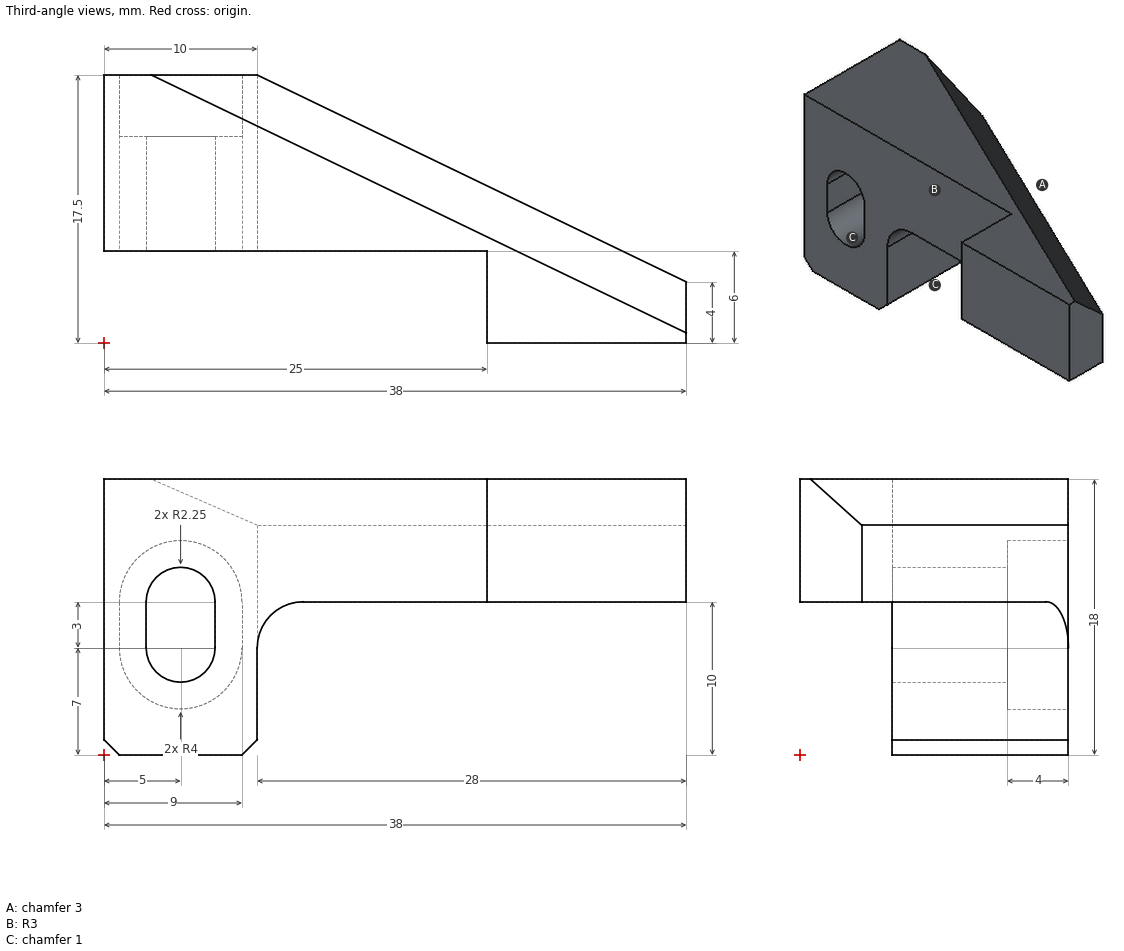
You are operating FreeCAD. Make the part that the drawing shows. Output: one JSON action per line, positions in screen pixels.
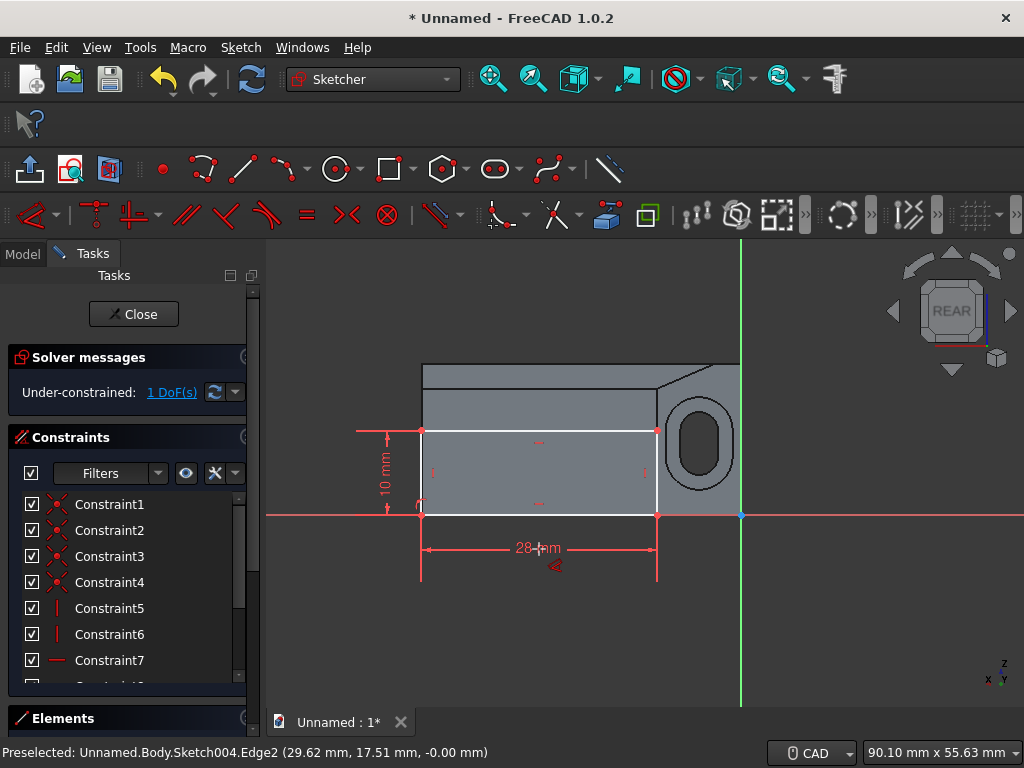
{"action": "left_click", "coordinate": [421, 431]}
{"action": "left_click", "coordinate": [655, 549]}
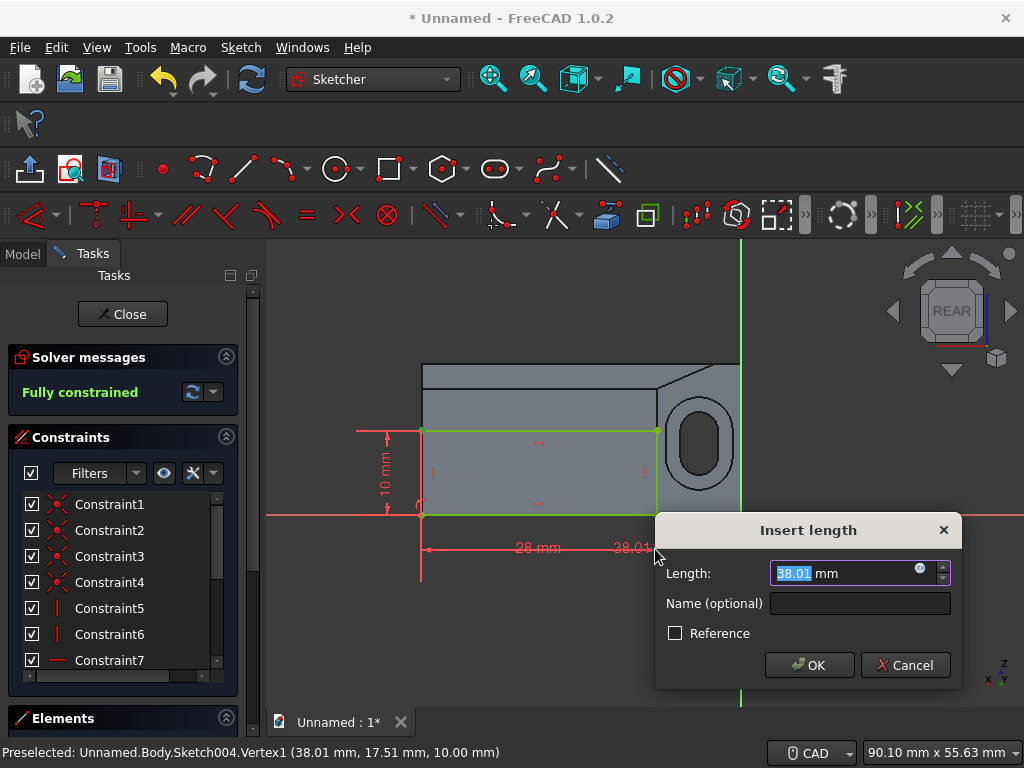
{"action": "type", "text": "38"}
{"action": "key", "text": "Return"}
{"action": "key", "text": "Escape"}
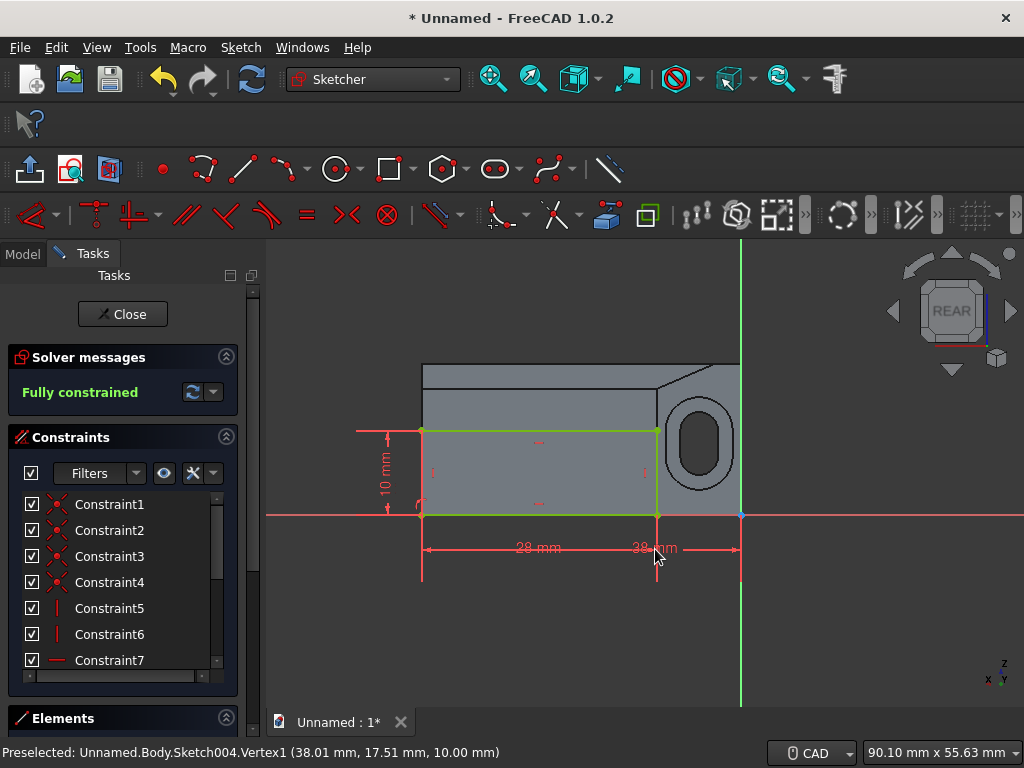
{"action": "left_click", "coordinate": [123, 314]}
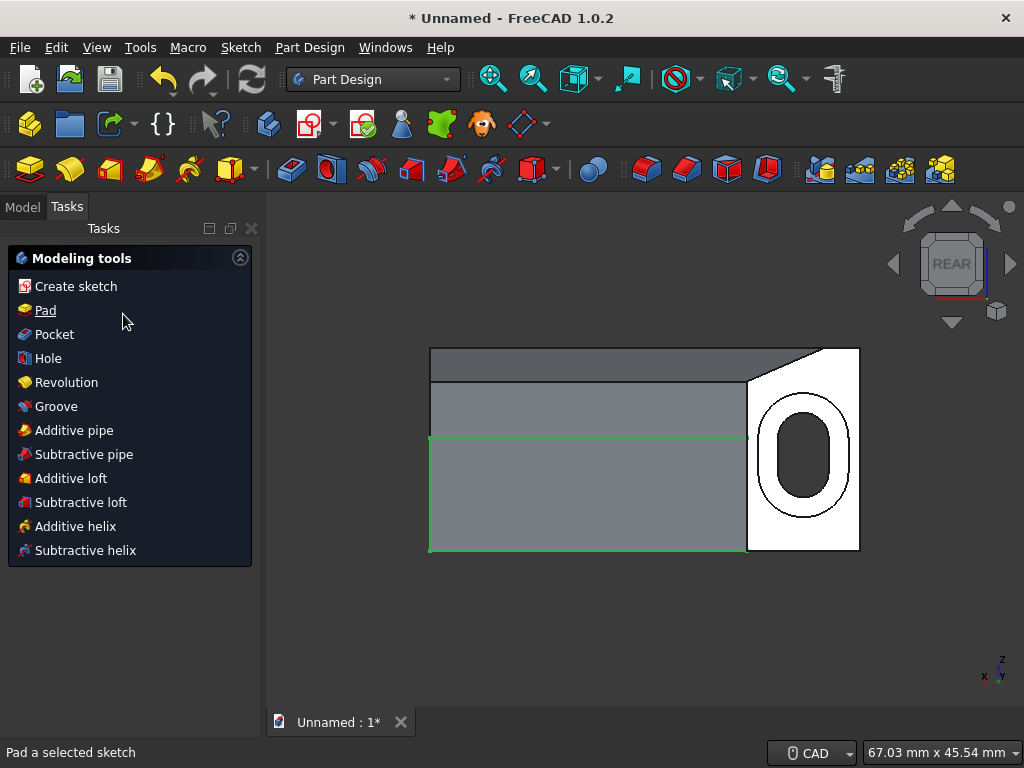
{"action": "left_click", "coordinate": [292, 170]}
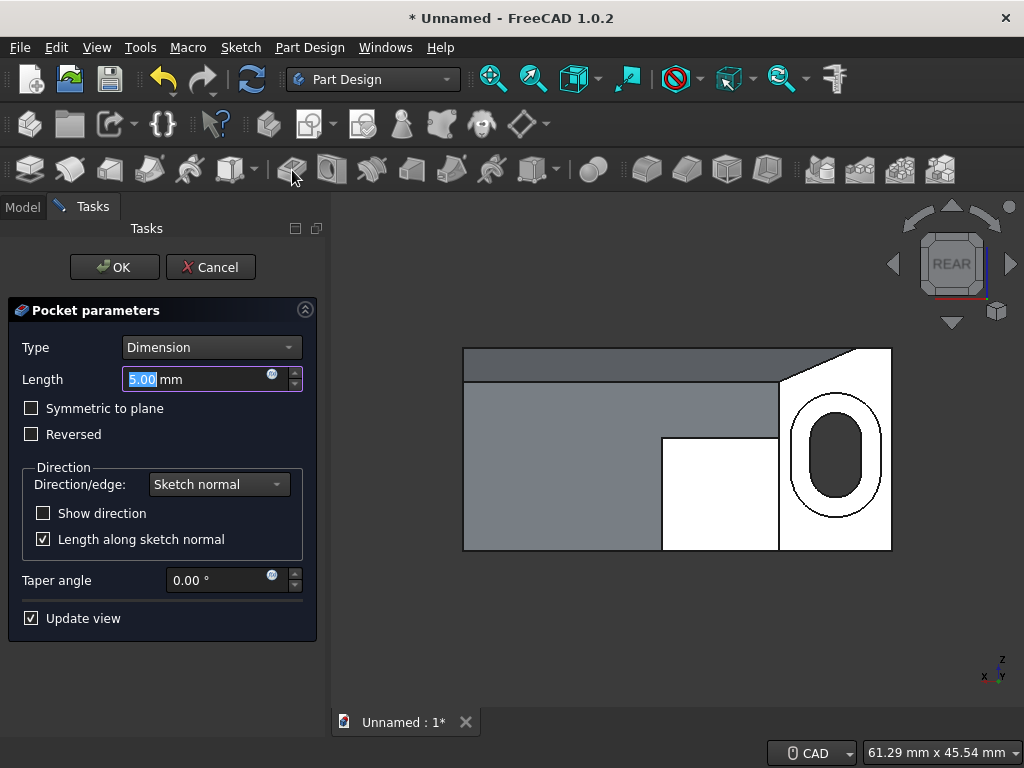
{"action": "left_click", "coordinate": [212, 348]}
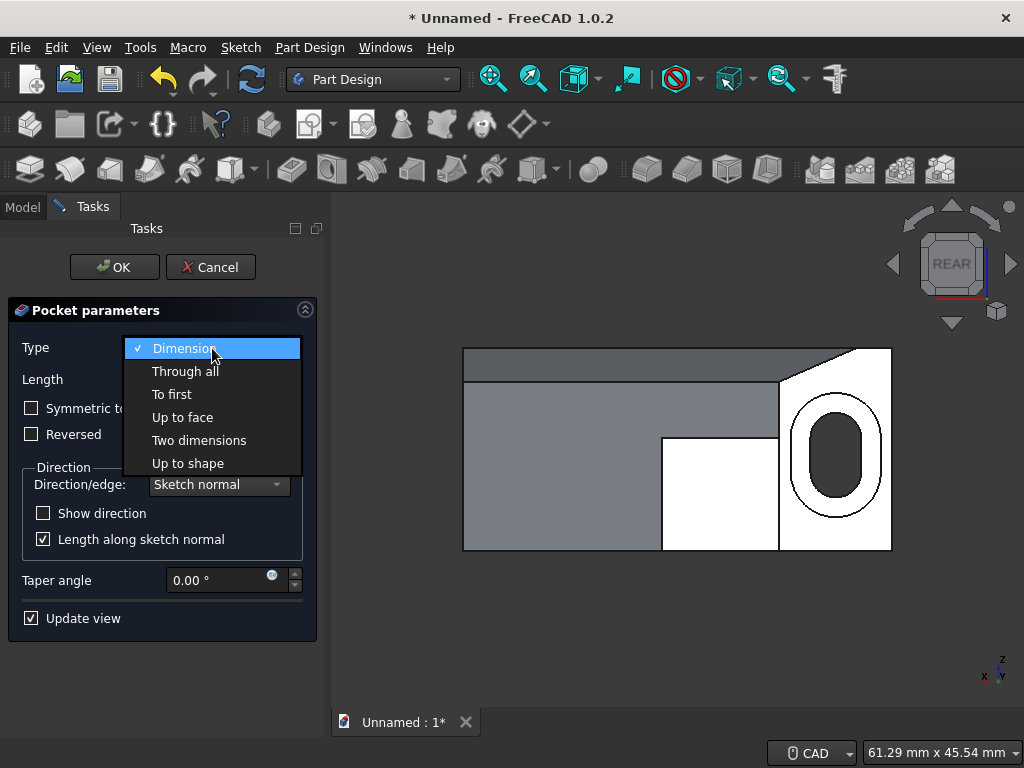
{"action": "left_click", "coordinate": [212, 372]}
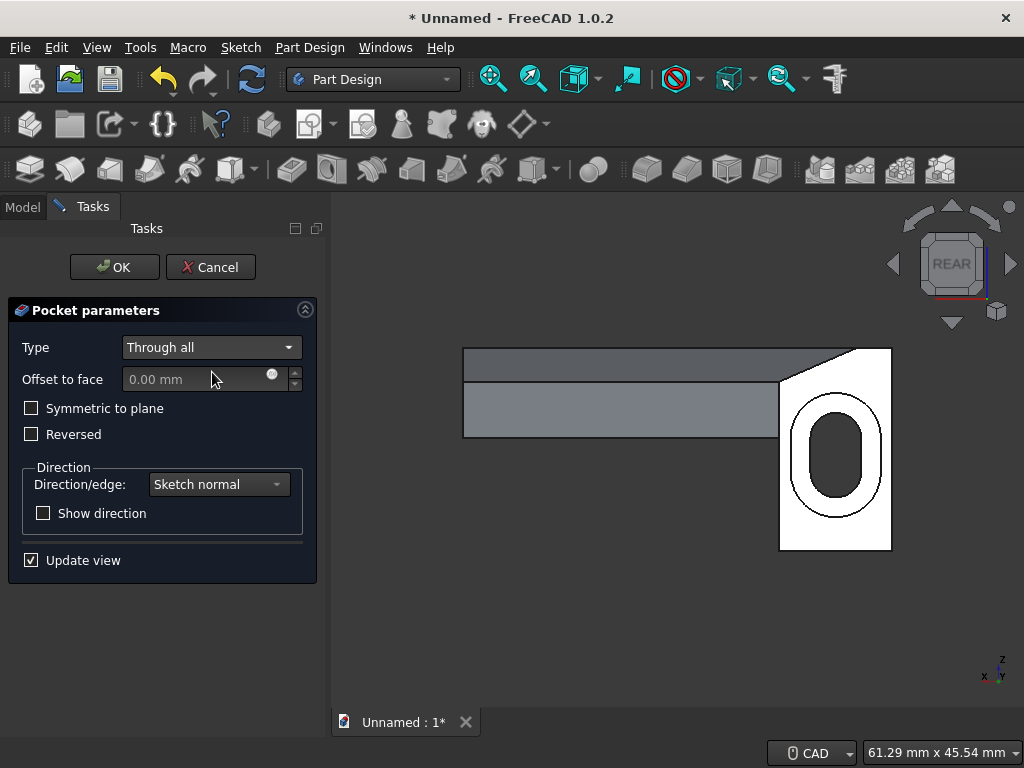
{"action": "left_click", "coordinate": [115, 267]}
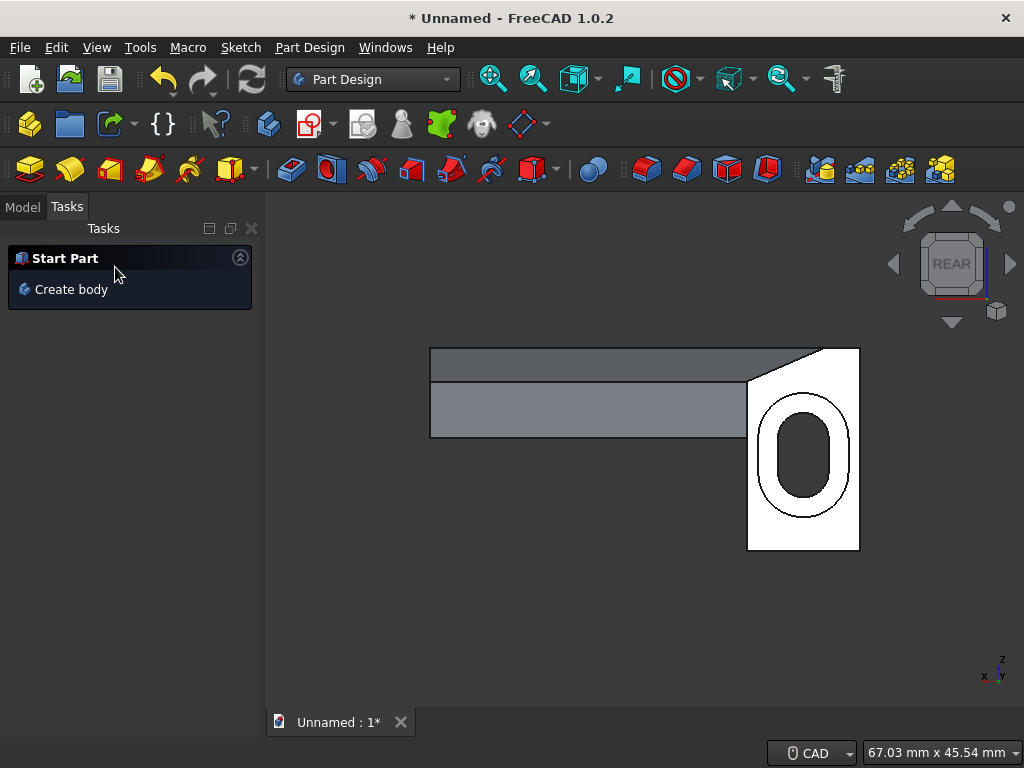
{"action": "key", "text": "0"}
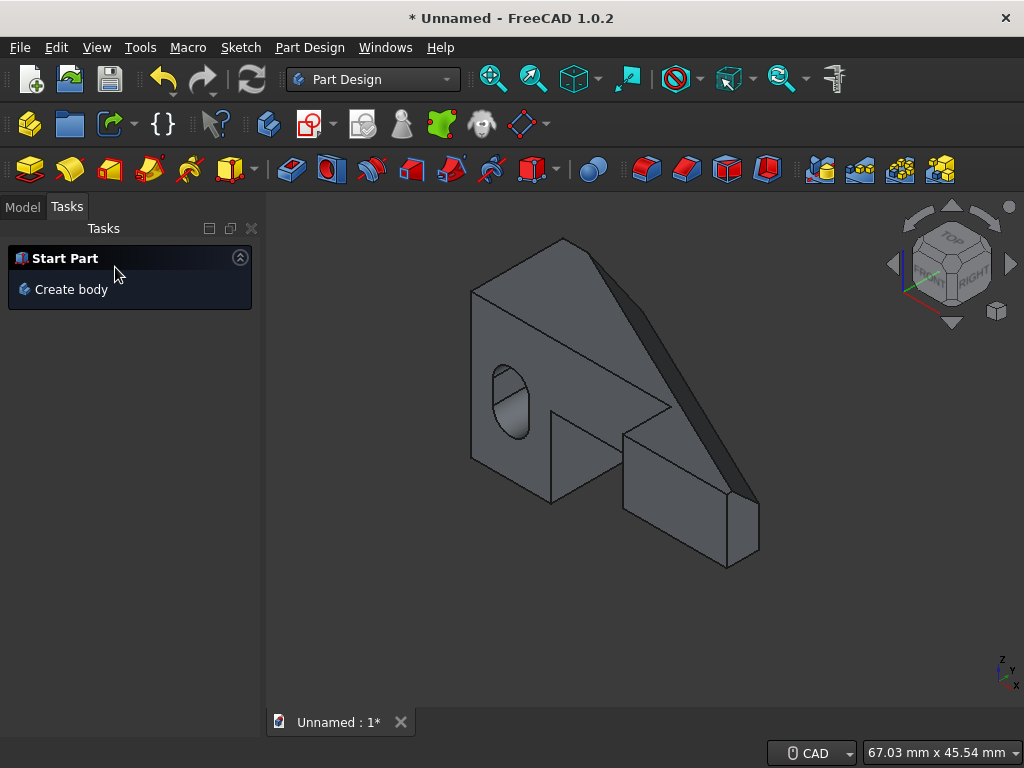
{"action": "key", "text": "2"}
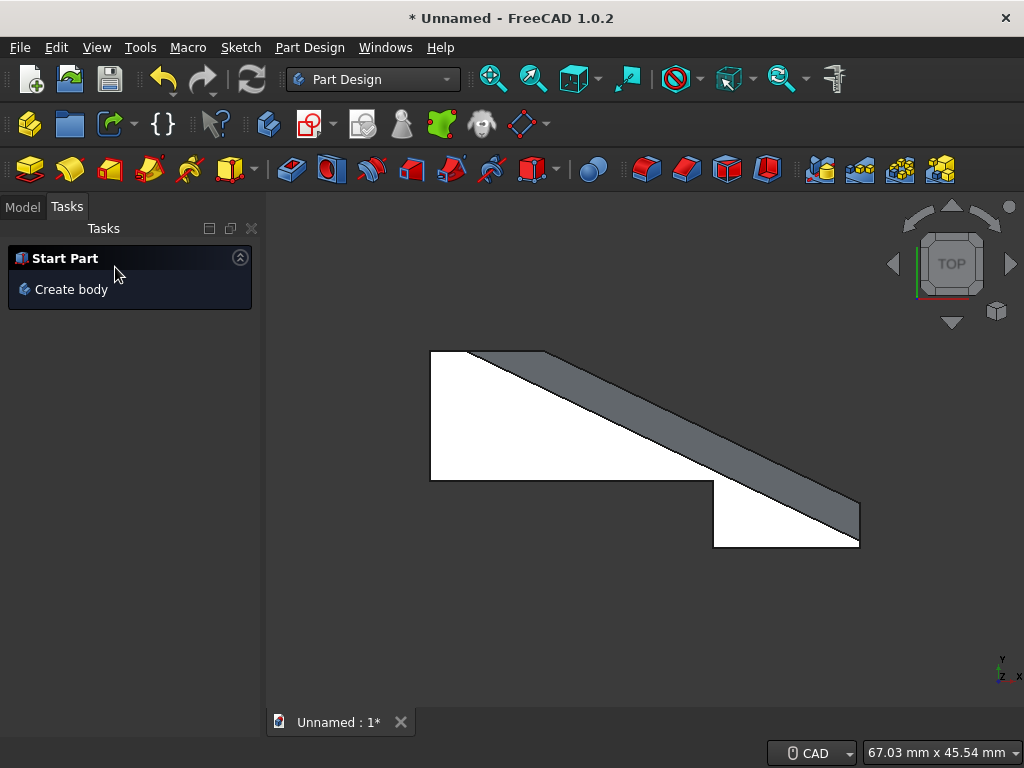
{"action": "key", "text": "1"}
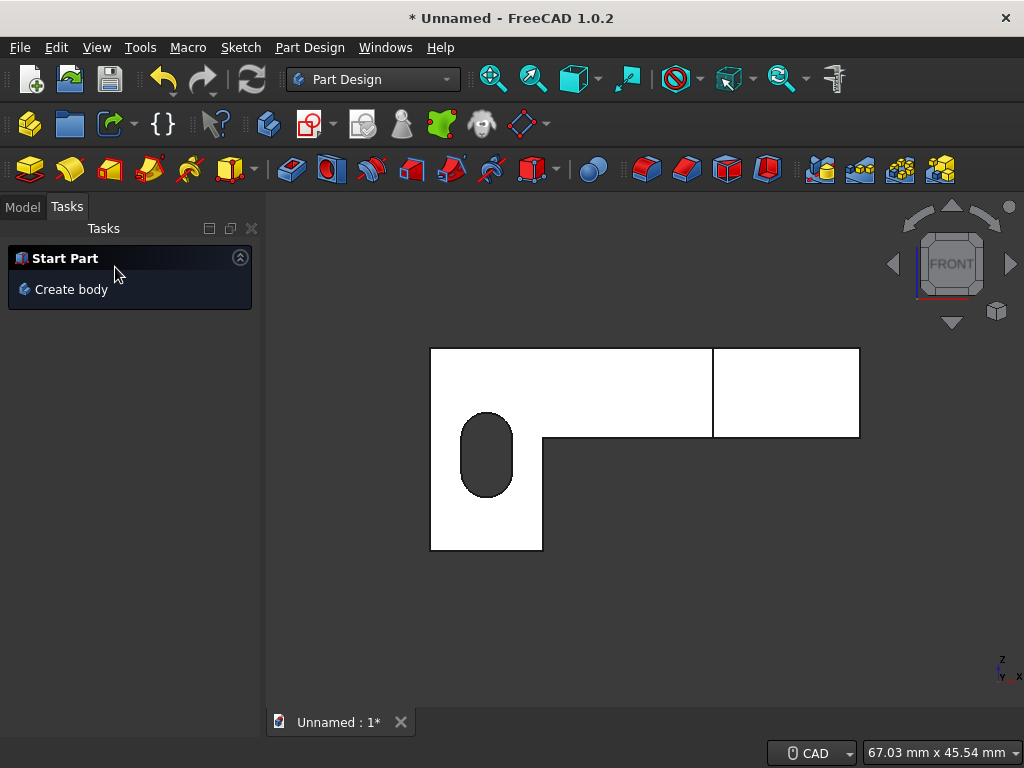
{"action": "key", "text": "3"}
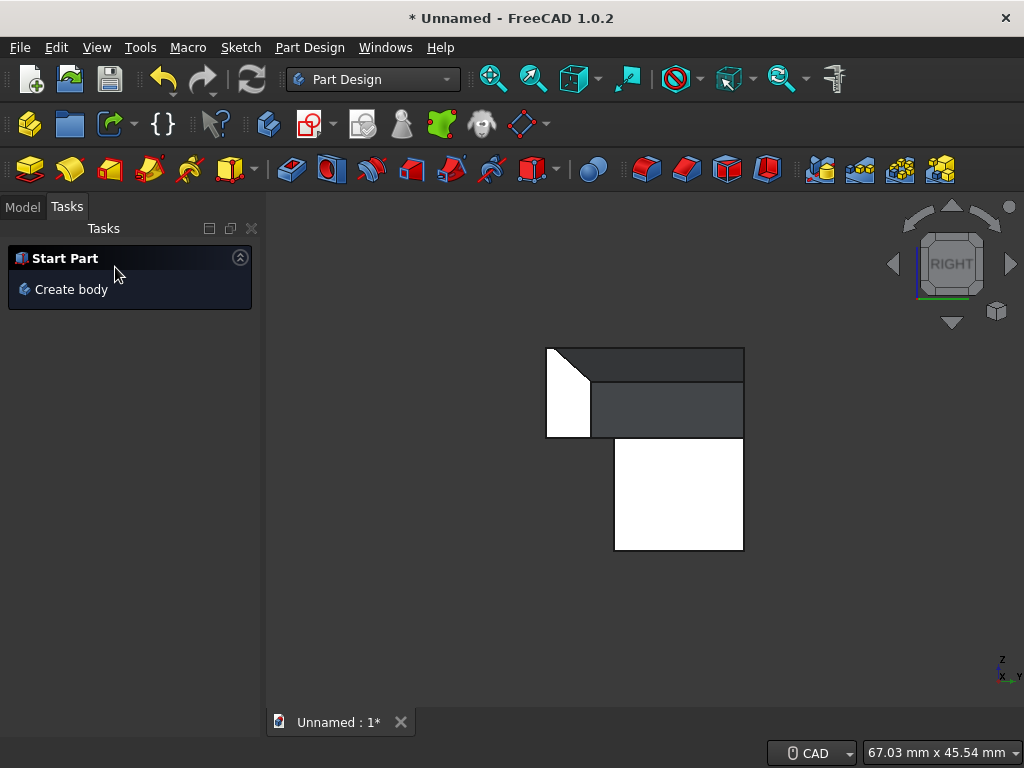
{"action": "key", "text": "v f"}